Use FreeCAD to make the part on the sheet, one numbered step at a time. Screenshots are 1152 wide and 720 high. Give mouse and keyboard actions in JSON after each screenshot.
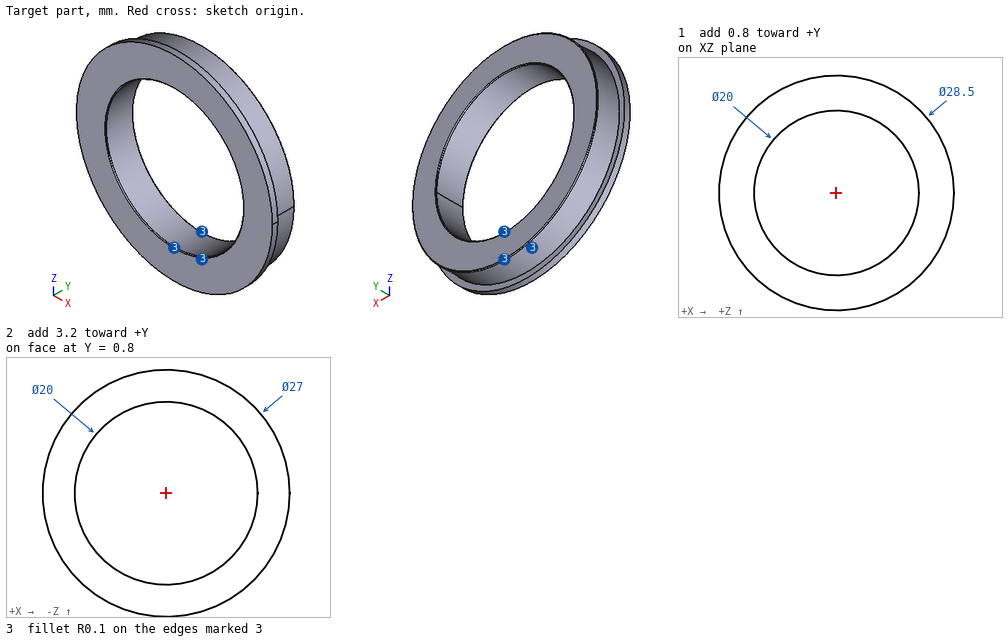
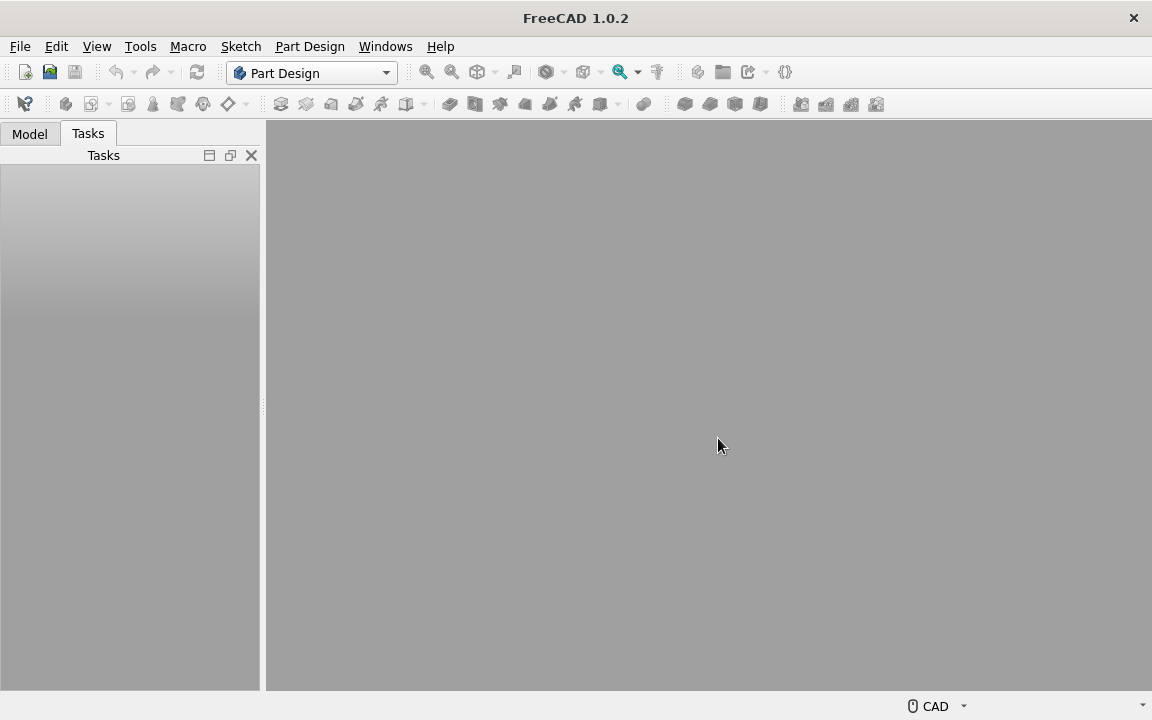
{"action": "key", "text": "ctrl+n"}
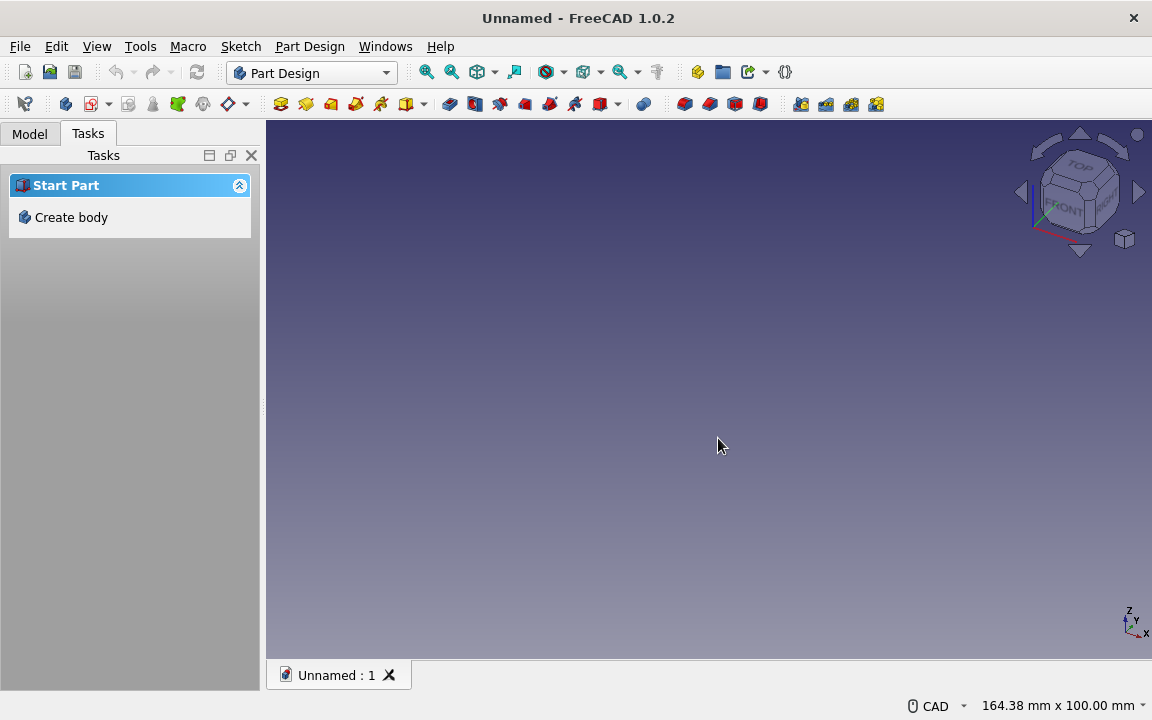
{"action": "left_click", "coordinate": [90, 104]}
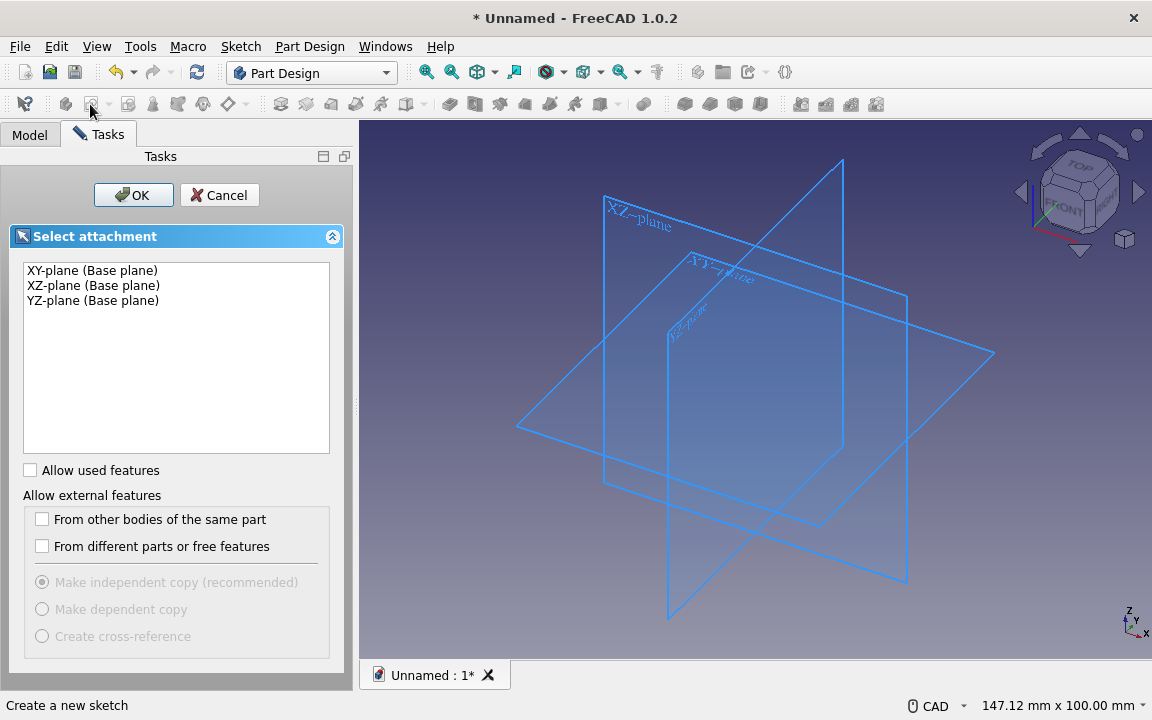
{"action": "left_click", "coordinate": [84, 286]}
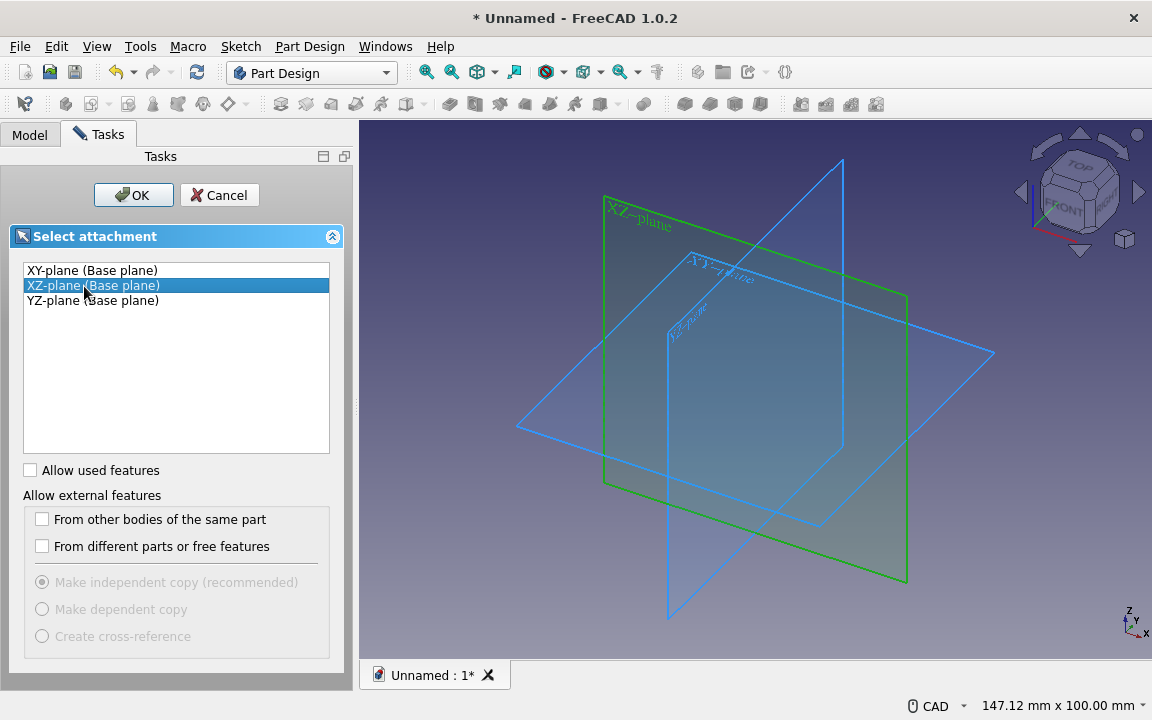
{"action": "left_click", "coordinate": [134, 195]}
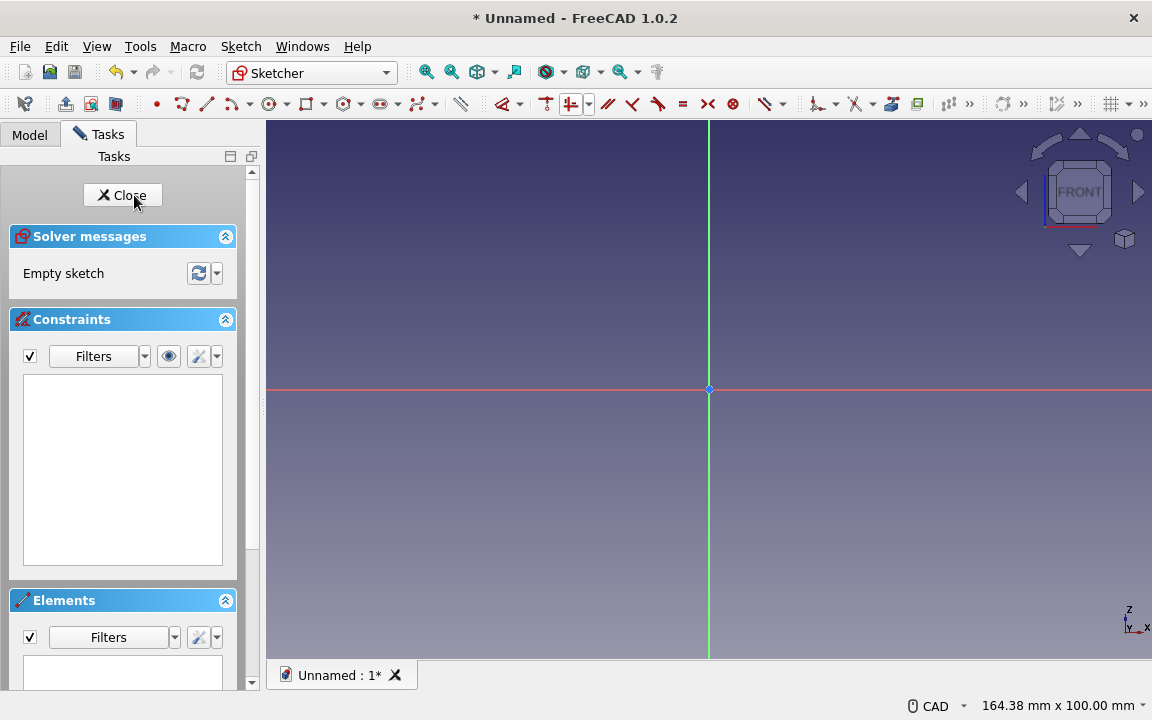
{"action": "scroll", "coordinate": [765, 390], "scroll_direction": "up", "scroll_amount": 4}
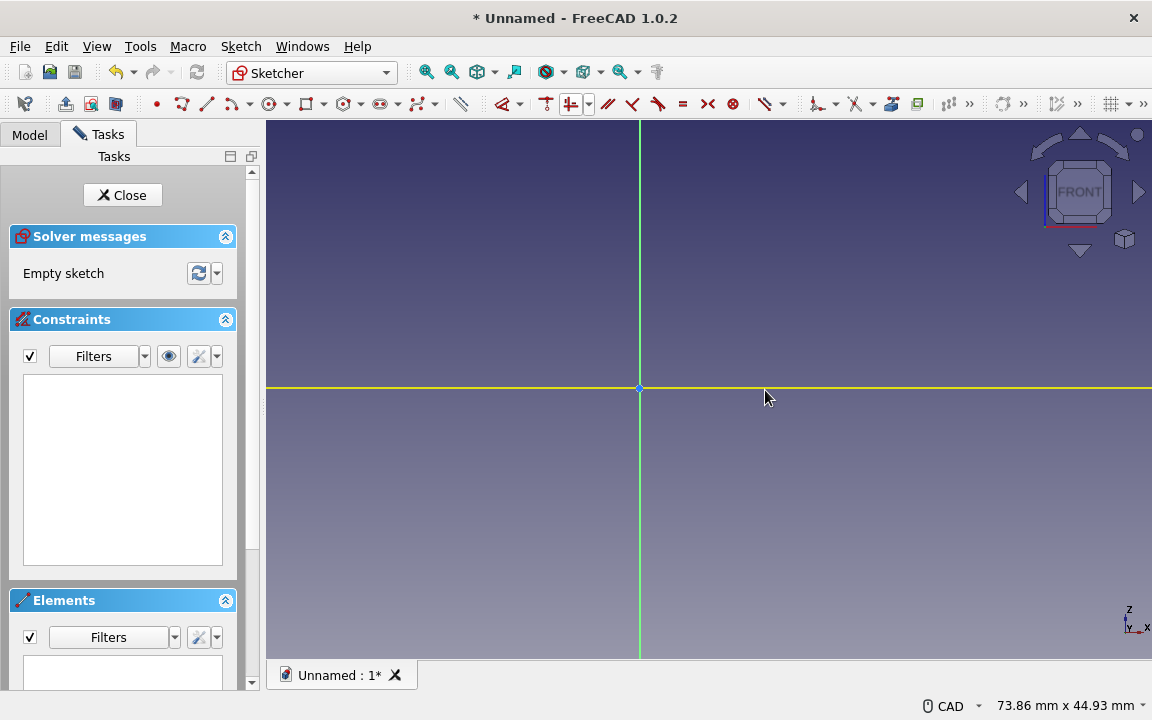
{"action": "key", "text": "g c"}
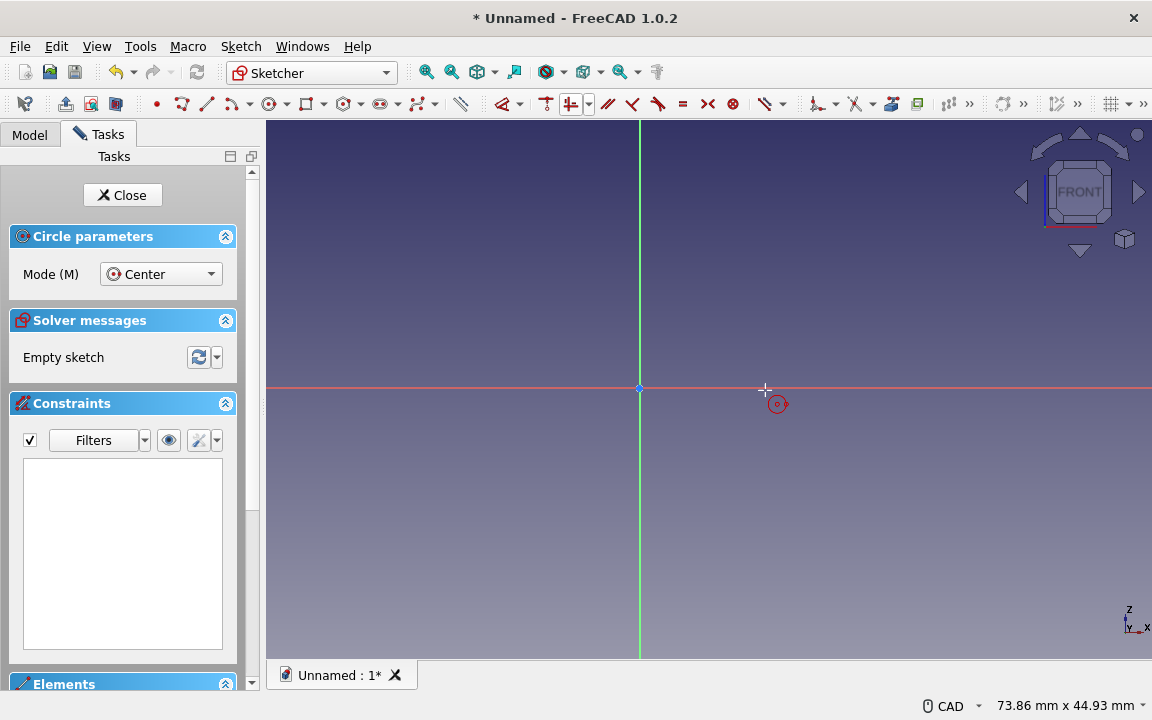
{"action": "left_click", "coordinate": [640, 388]}
{"action": "mouse_move", "coordinate": [761, 267]}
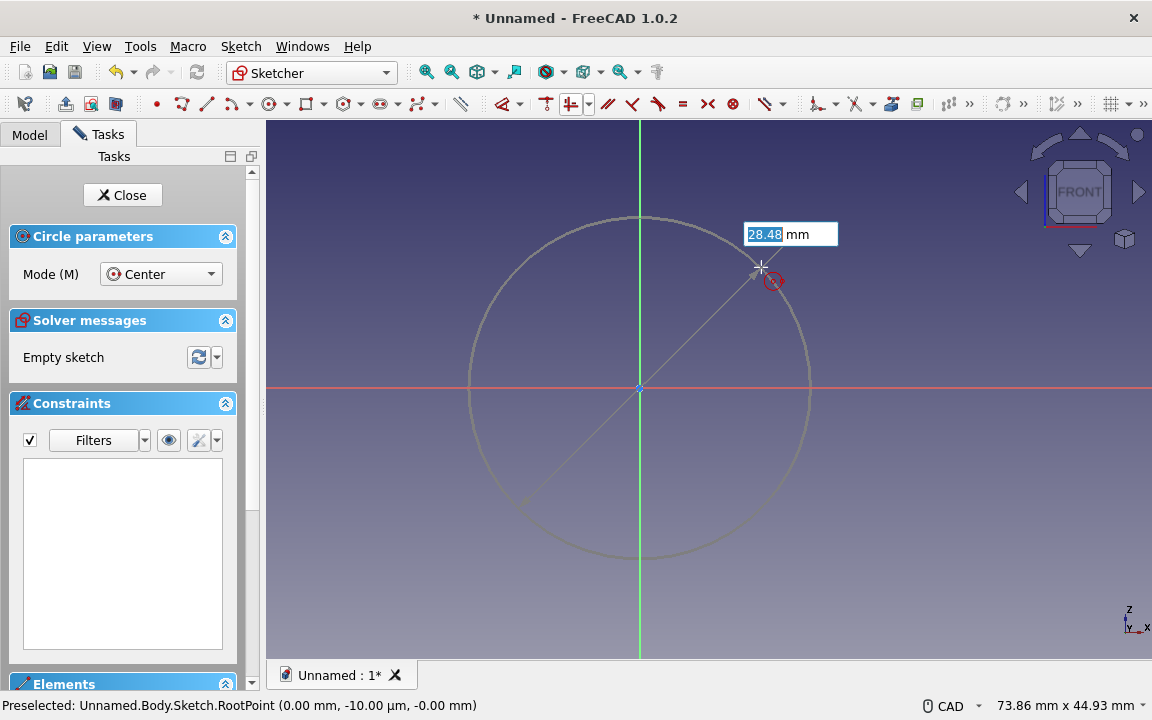
{"action": "type", "text": "28.5"}
{"action": "key", "text": "Return"}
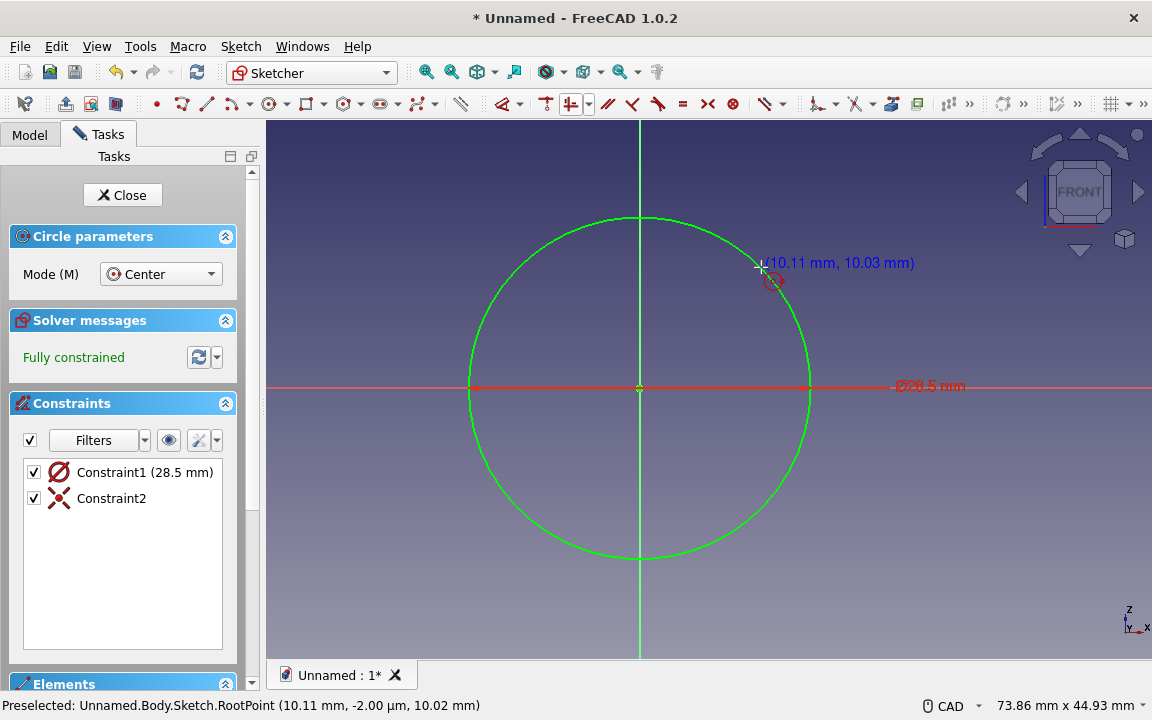
{"action": "left_click", "coordinate": [640, 388]}
{"action": "mouse_move", "coordinate": [725, 303]}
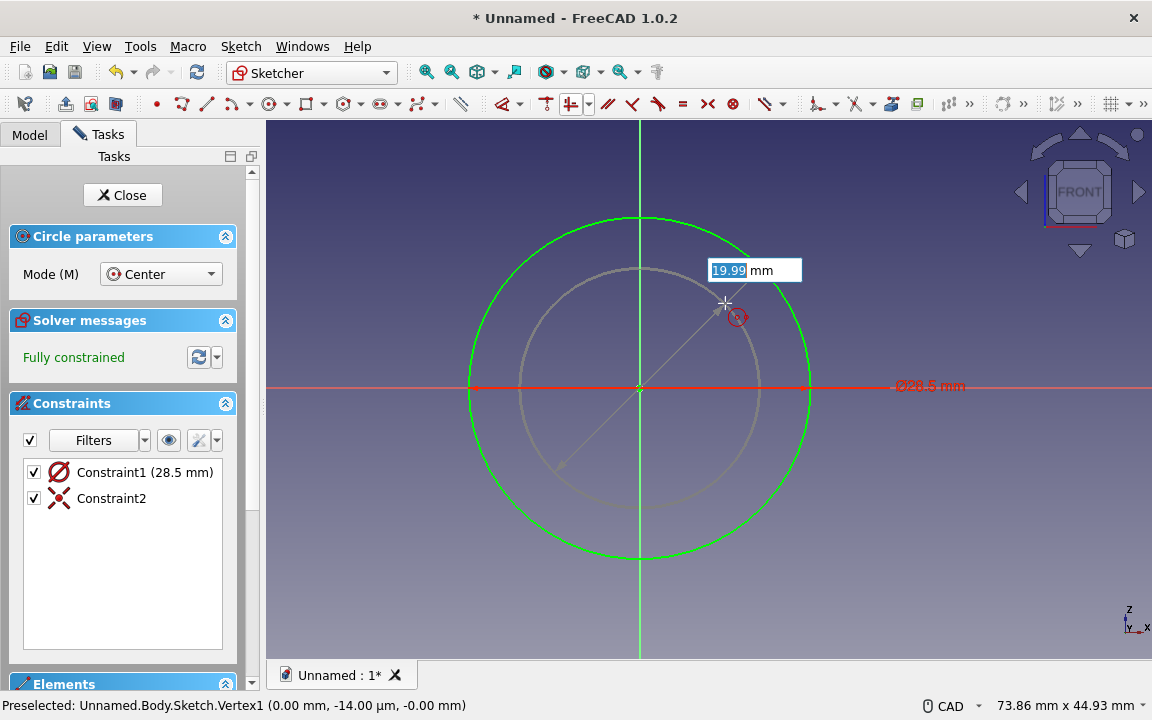
{"action": "type", "text": "20"}
{"action": "key", "text": "Return"}
{"action": "key", "text": "Escape"}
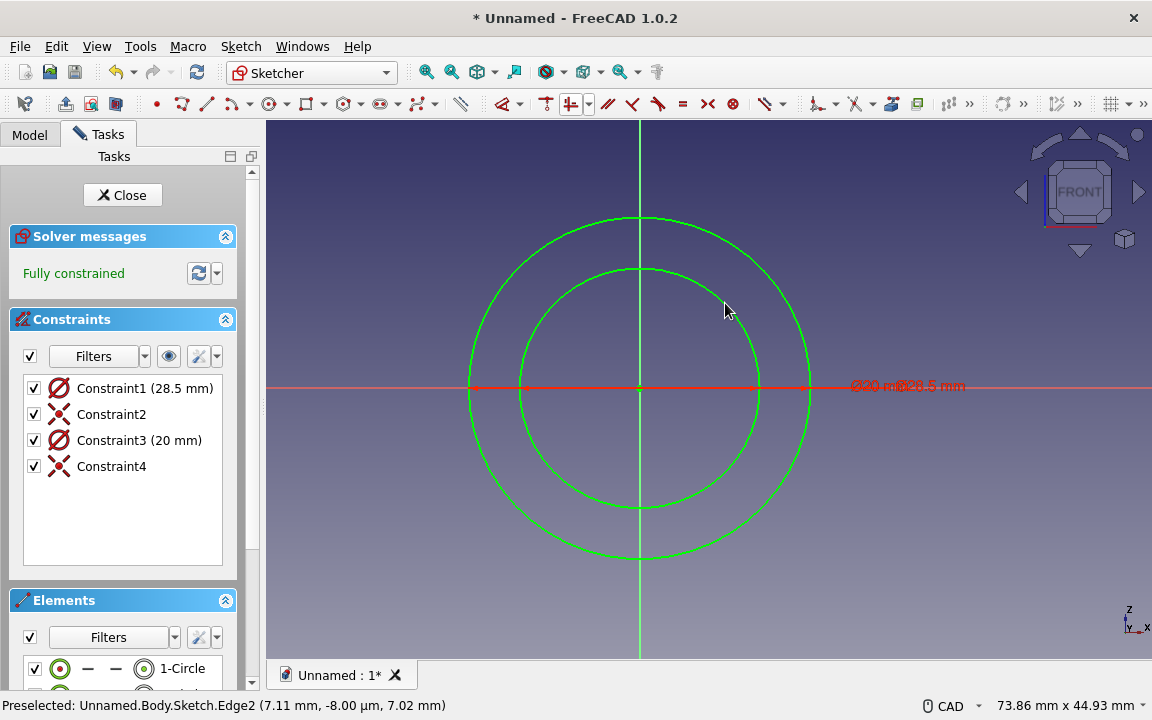
{"action": "left_click", "coordinate": [123, 195]}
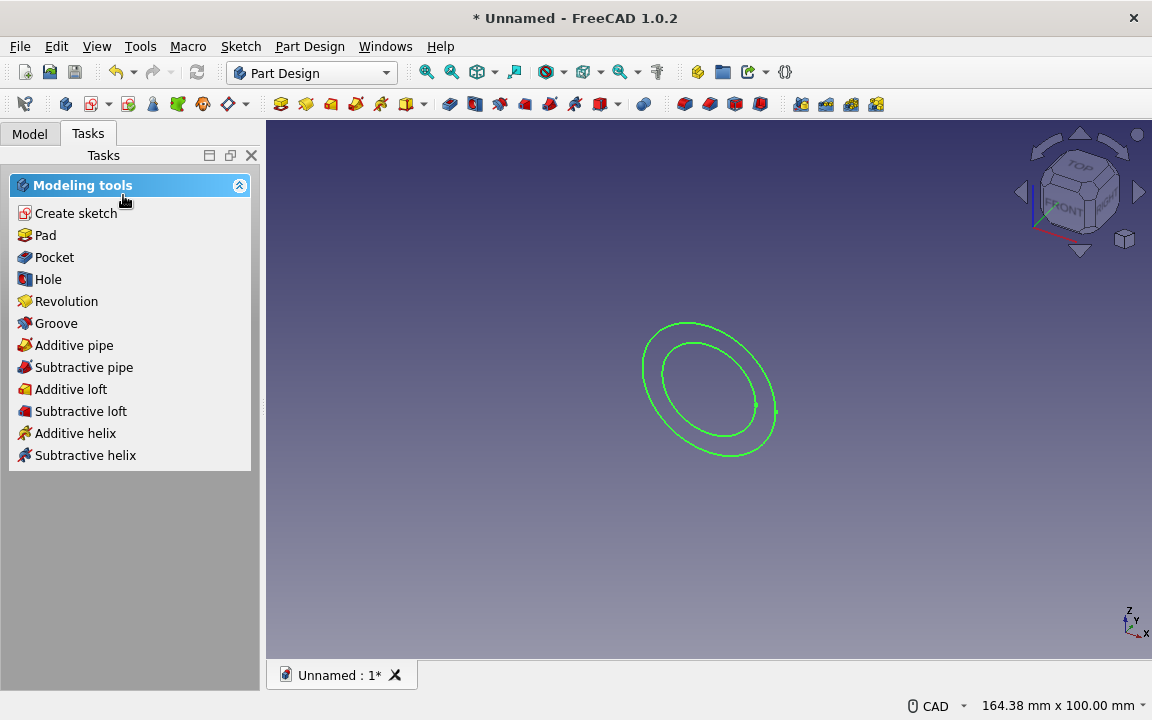
{"action": "left_click", "coordinate": [281, 104]}